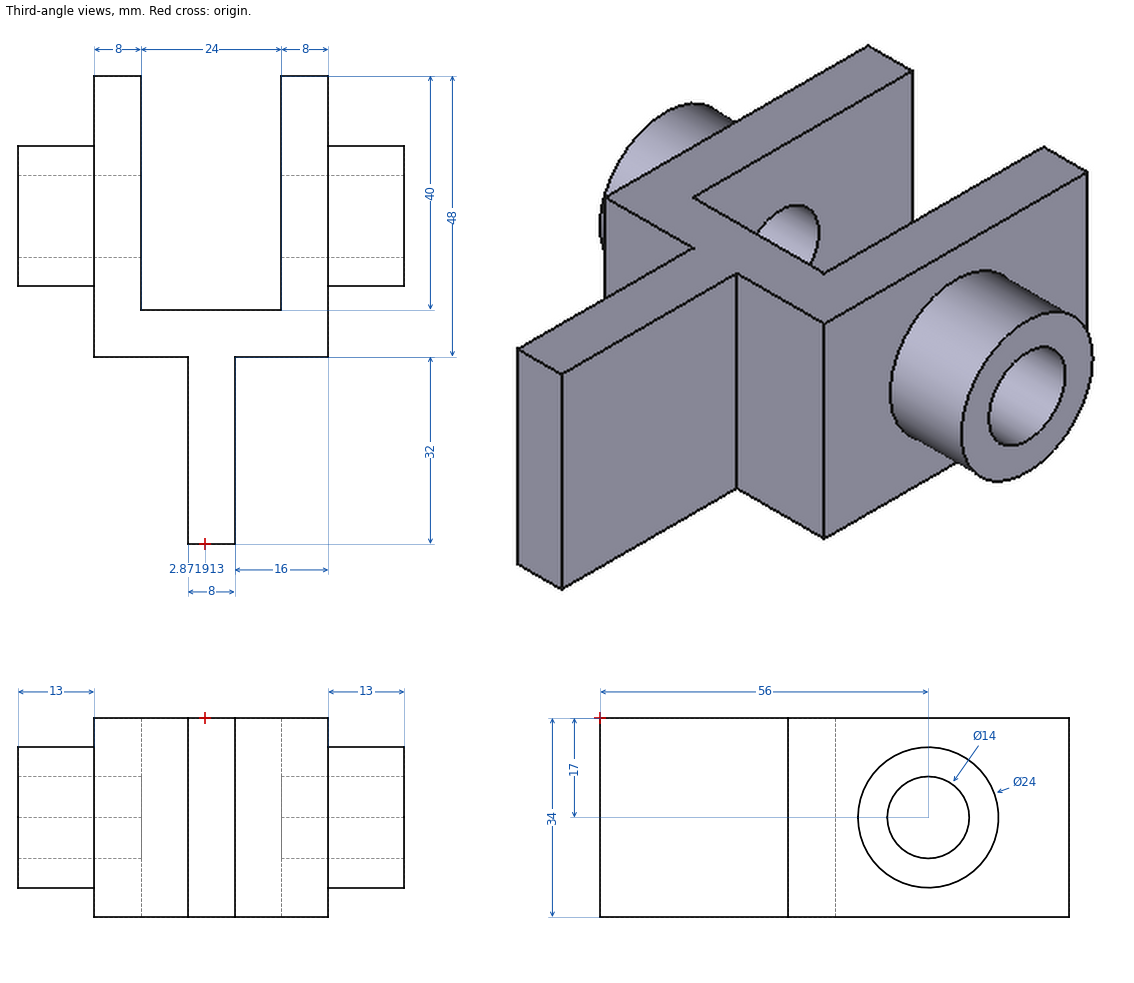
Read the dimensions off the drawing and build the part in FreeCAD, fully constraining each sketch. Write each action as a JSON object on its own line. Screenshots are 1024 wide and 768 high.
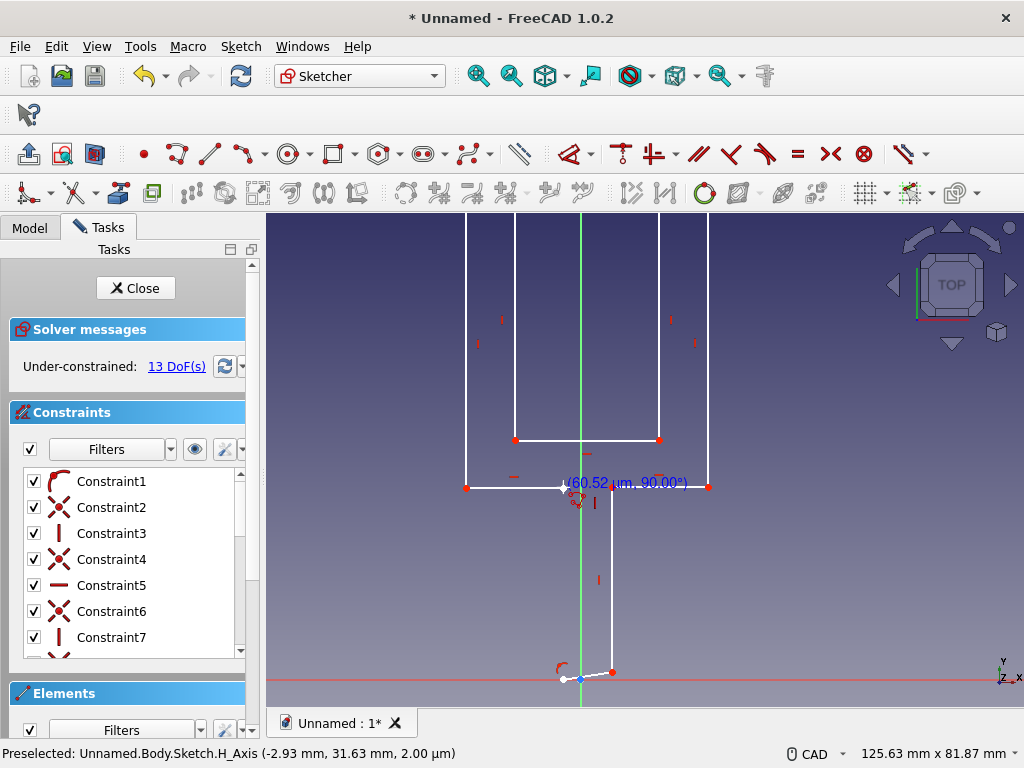
{"action": "scroll", "coordinate": [554, 504], "scroll_direction": "down", "scroll_amount": 2}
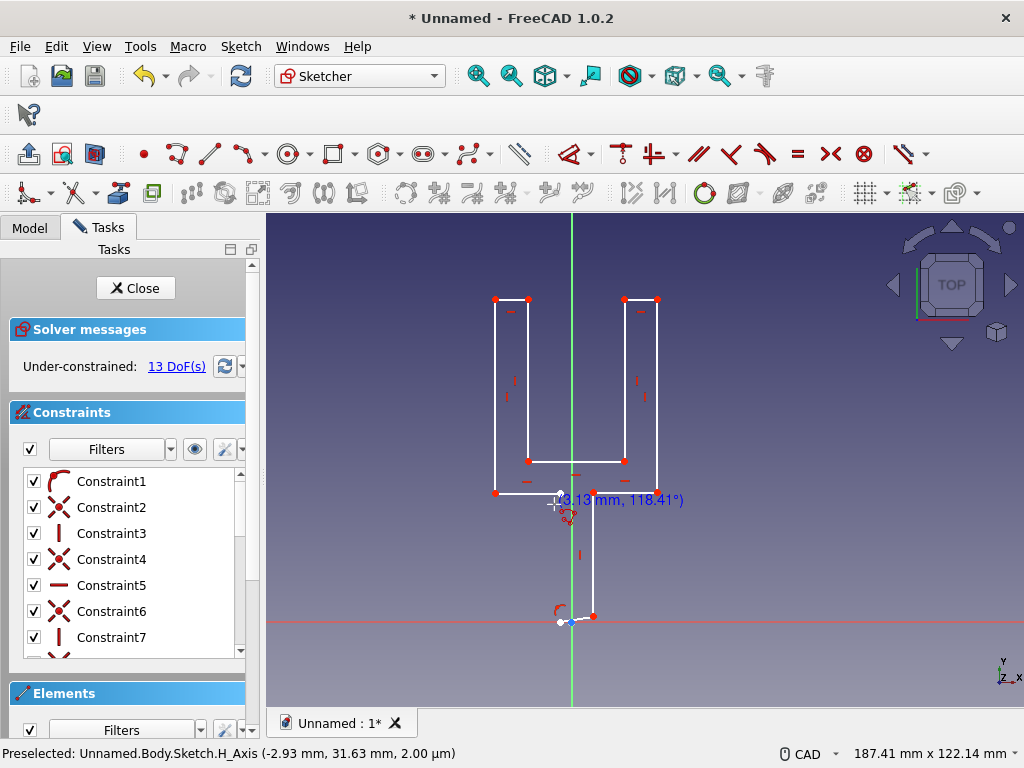
{"action": "scroll", "coordinate": [560, 622], "scroll_direction": "up", "scroll_amount": 2}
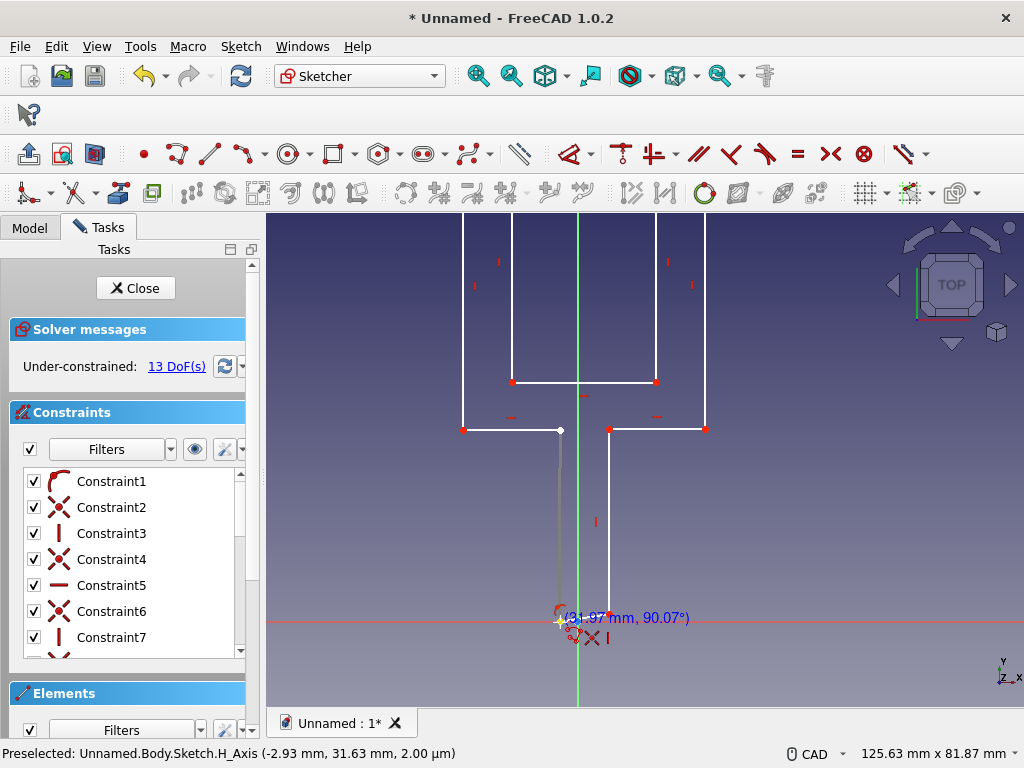
{"action": "left_click", "coordinate": [560, 622]}
{"action": "key", "text": "Escape"}
{"action": "key", "text": "Escape"}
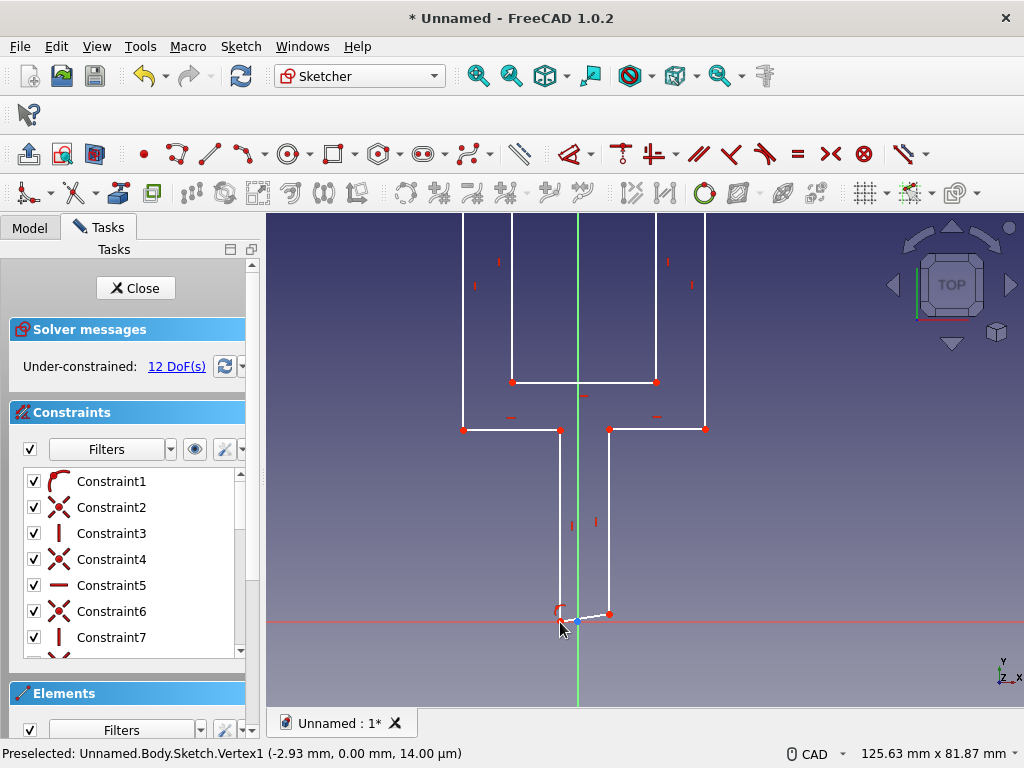
{"action": "left_click", "coordinate": [570, 620]}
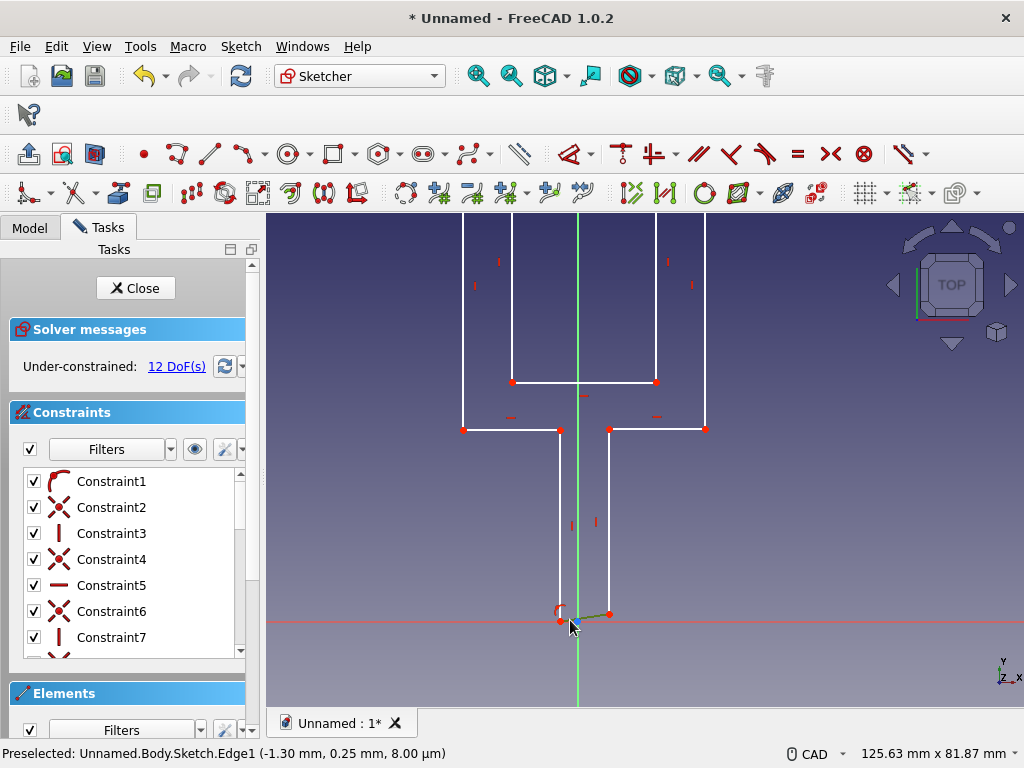
{"action": "key", "text": "h"}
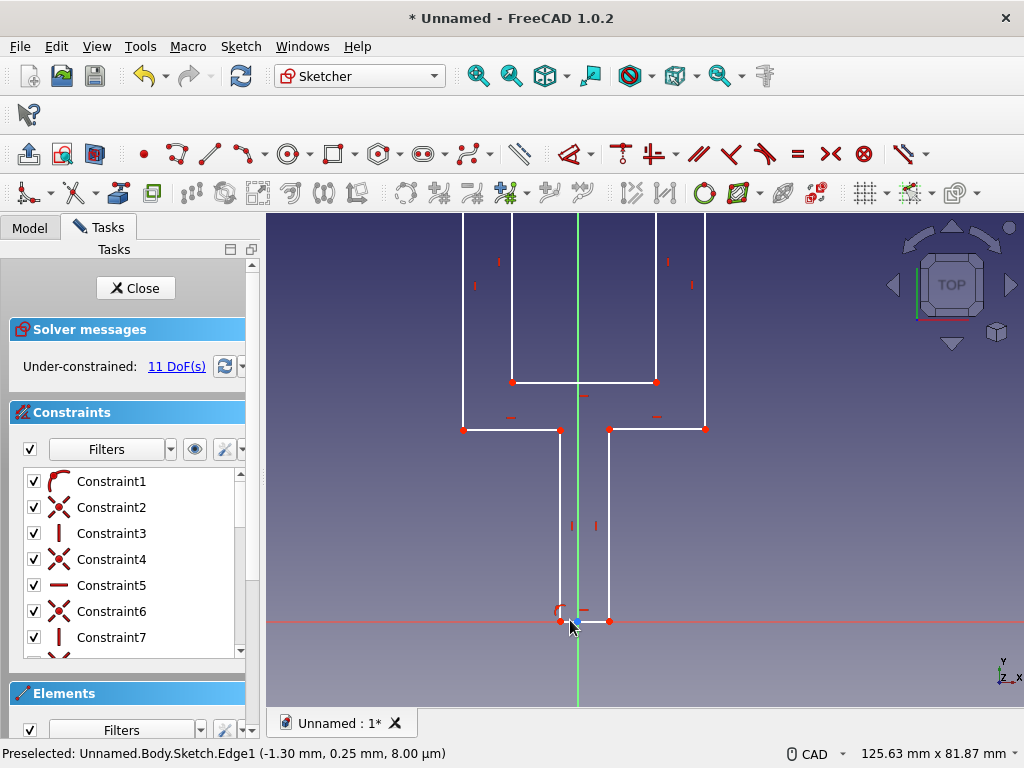
{"action": "key", "text": "d"}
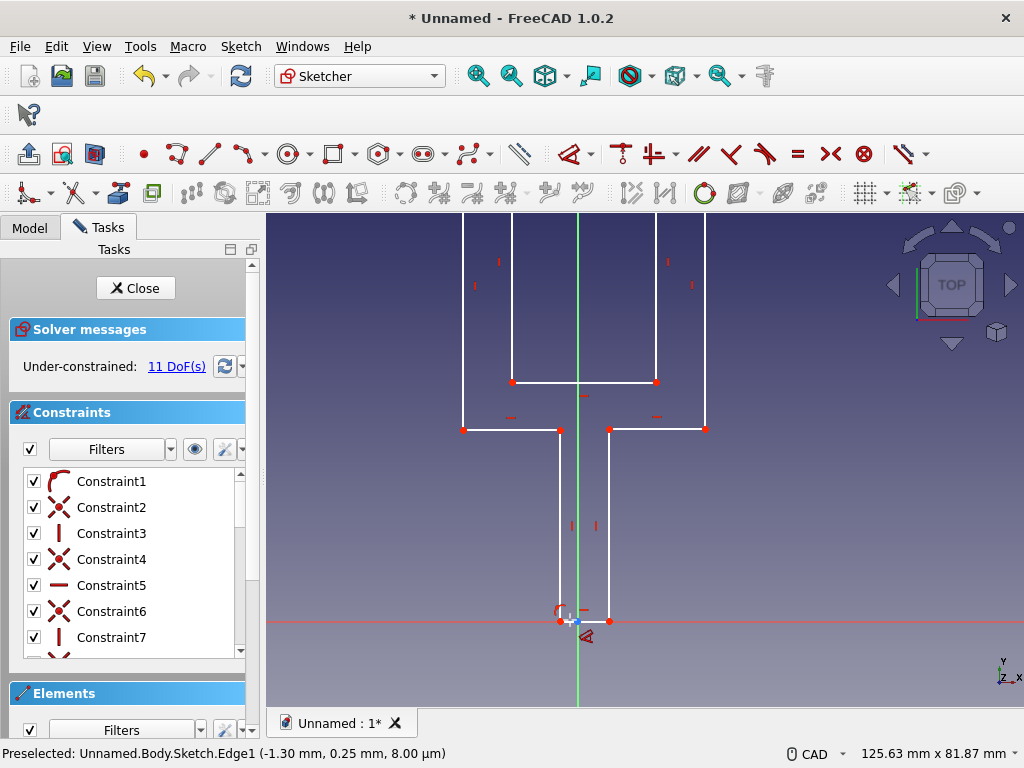
{"action": "left_click", "coordinate": [594, 622]}
{"action": "left_click", "coordinate": [596, 656]}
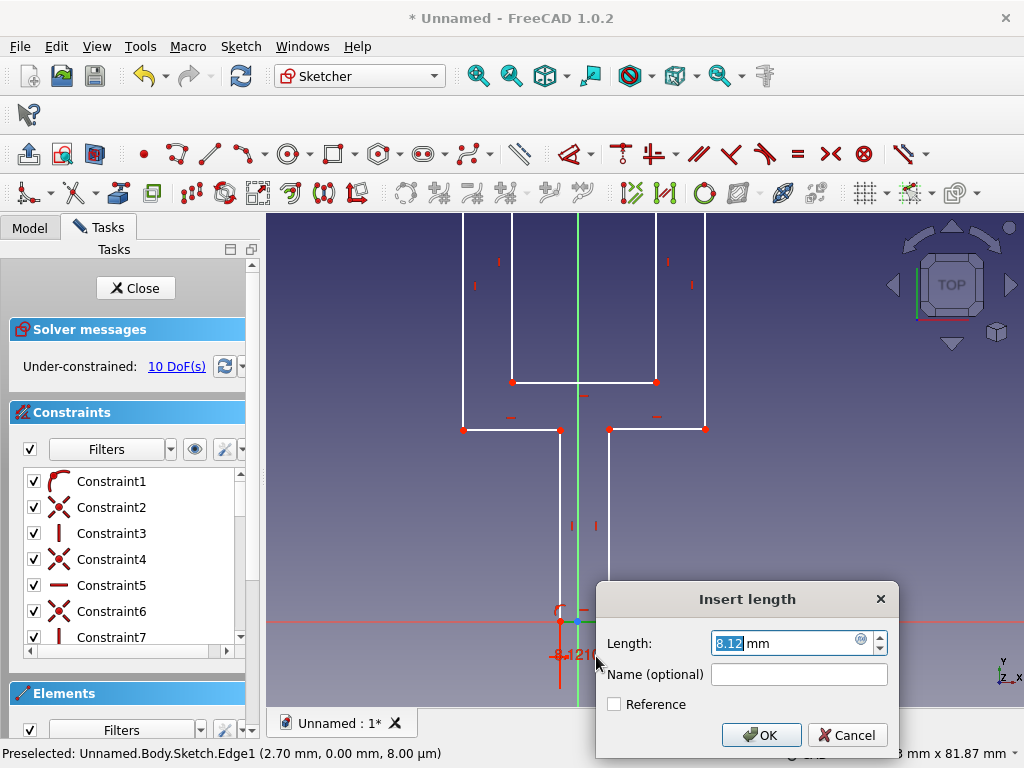
{"action": "type", "text": "8"}
{"action": "key", "text": "Return"}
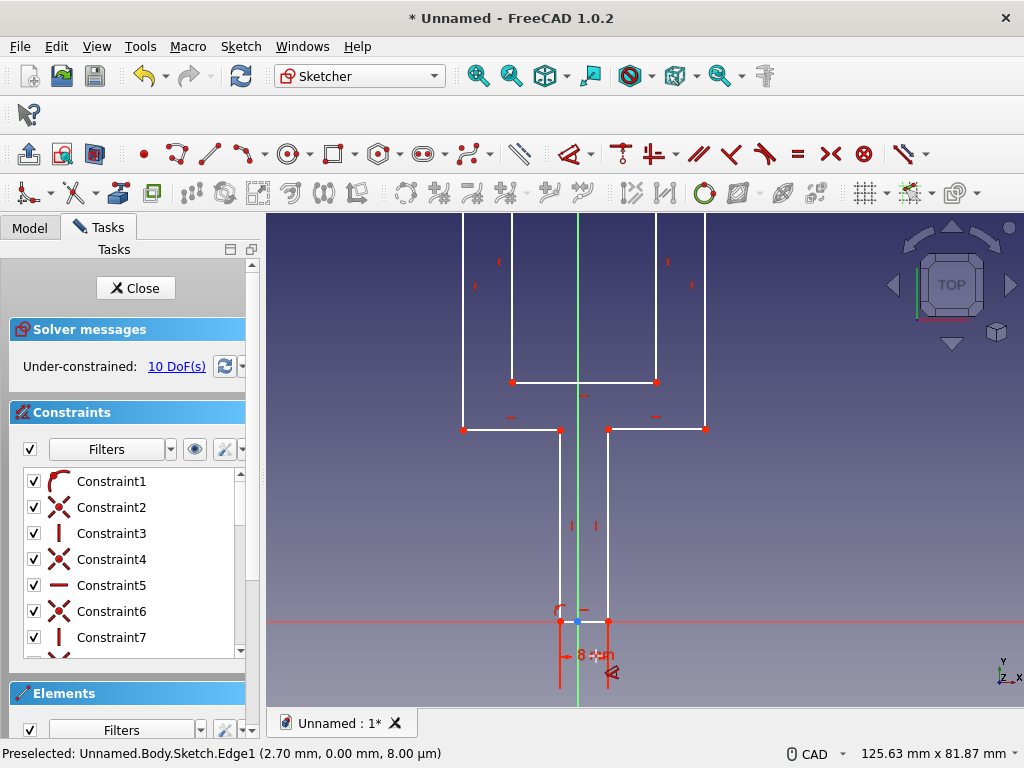
{"action": "scroll", "coordinate": [560, 622], "scroll_direction": "down", "scroll_amount": 2}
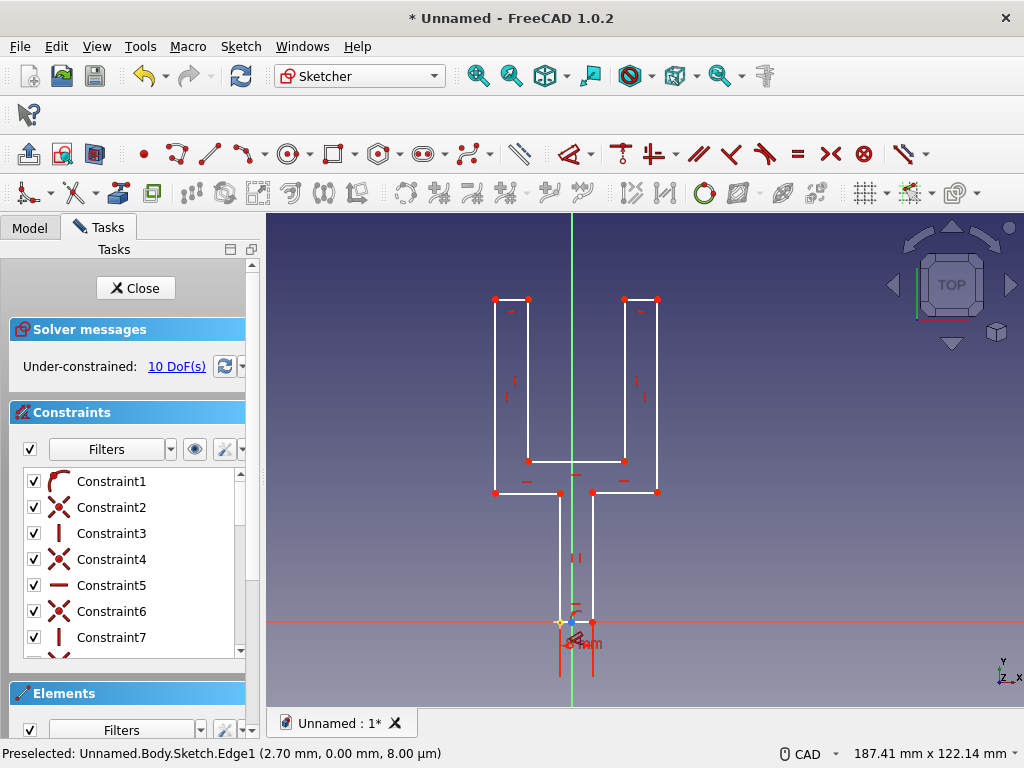
{"action": "scroll", "coordinate": [648, 300], "scroll_direction": "up", "scroll_amount": 2}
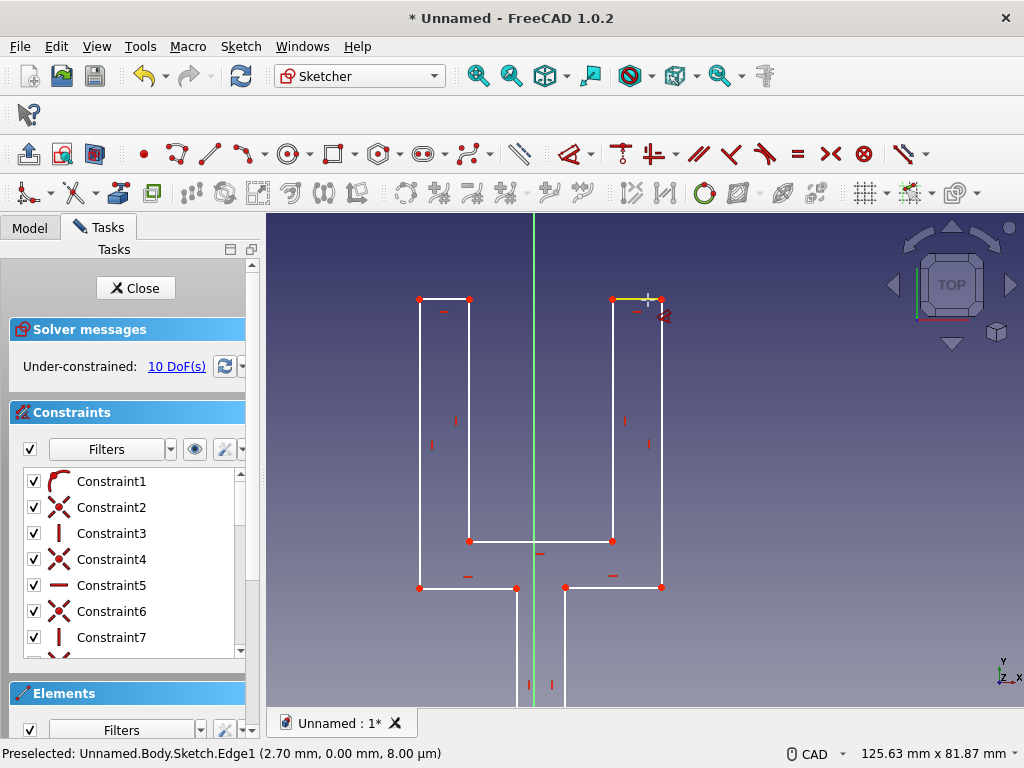
{"action": "left_click", "coordinate": [647, 299]}
{"action": "left_click", "coordinate": [637, 265]}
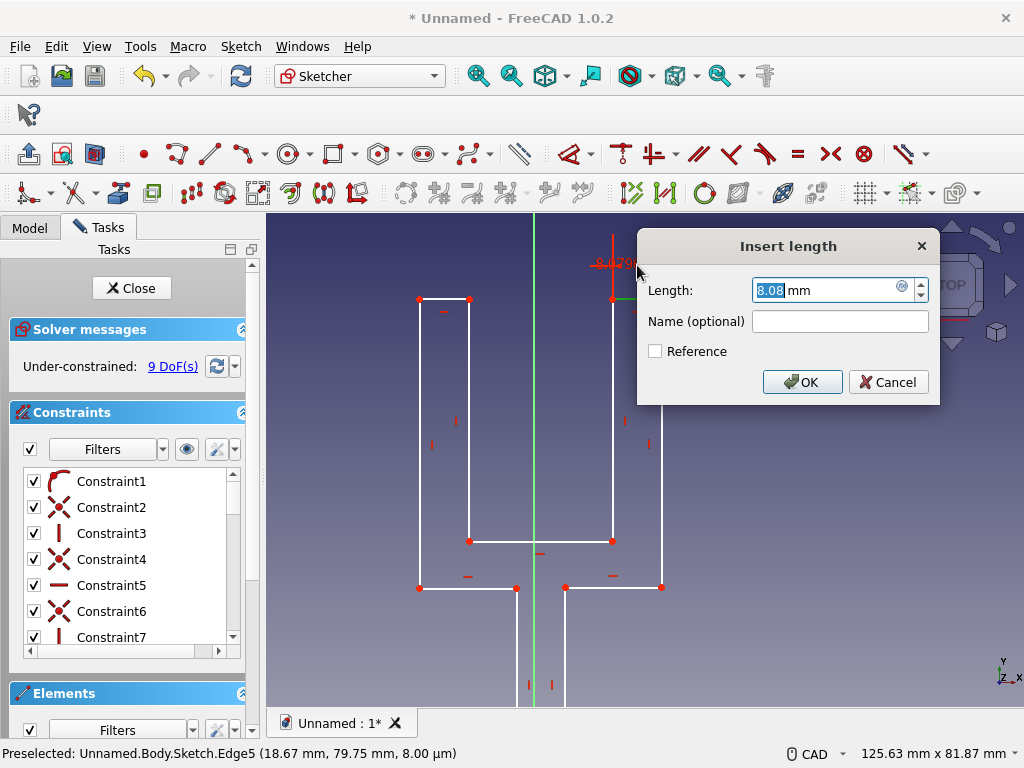
{"action": "type", "text": "8"}
{"action": "key", "text": "Return"}